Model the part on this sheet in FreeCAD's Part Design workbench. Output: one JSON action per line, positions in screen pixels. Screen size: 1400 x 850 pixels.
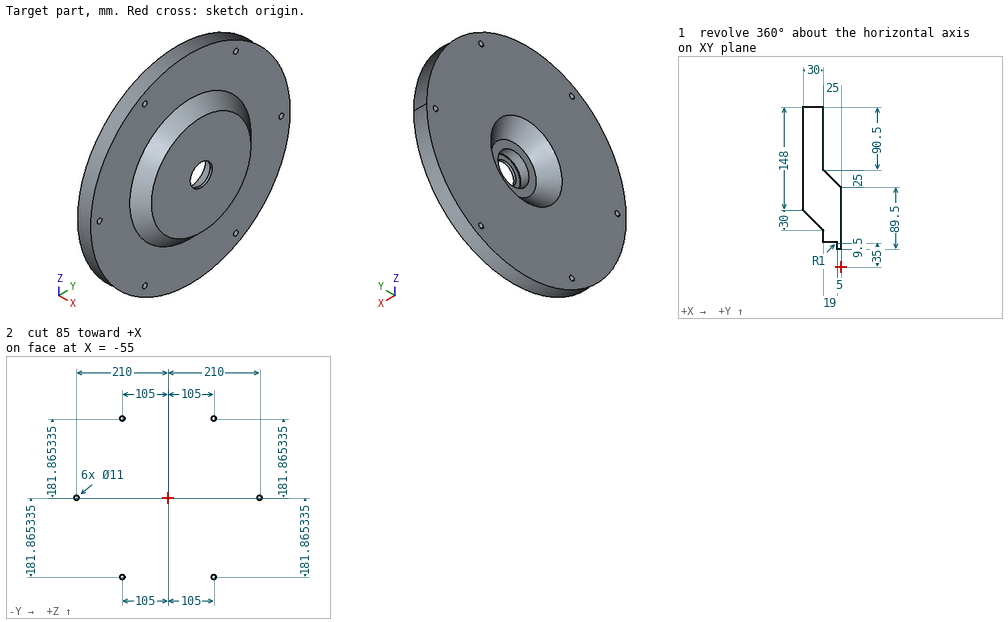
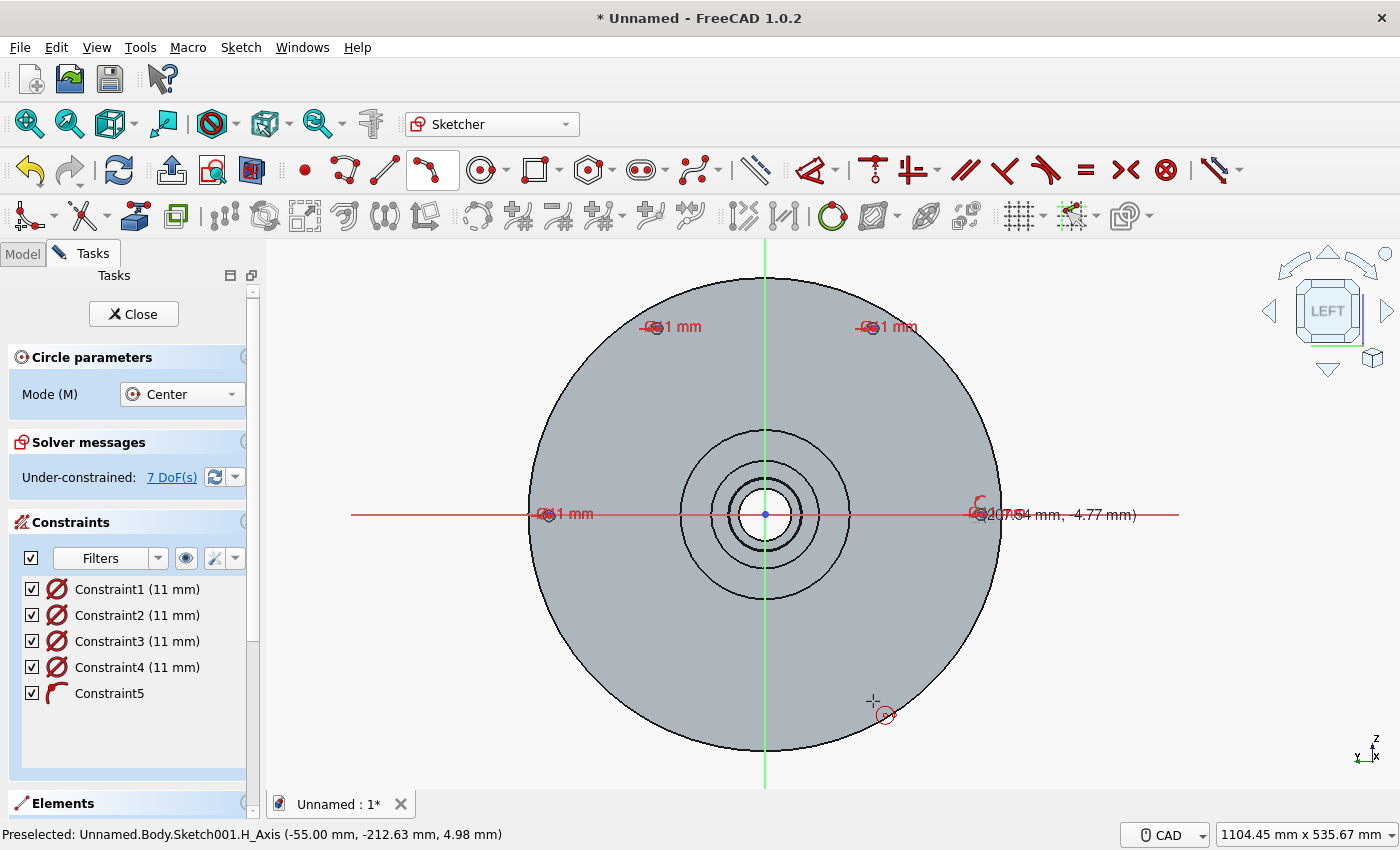
{"action": "left_click", "coordinate": [873, 701]}
{"action": "mouse_move", "coordinate": [877, 697]}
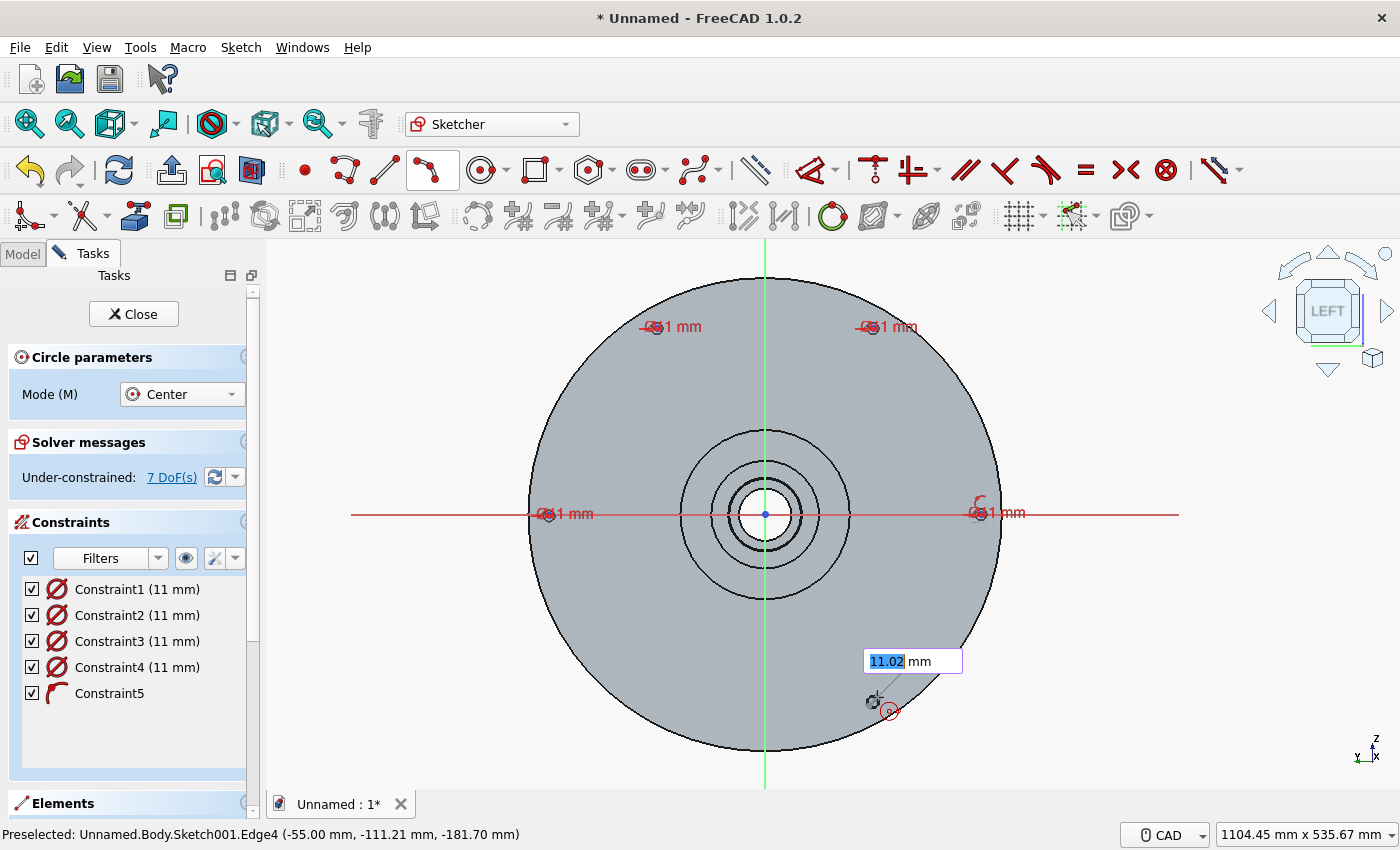
{"action": "type", "text": "11"}
{"action": "key", "text": "Return"}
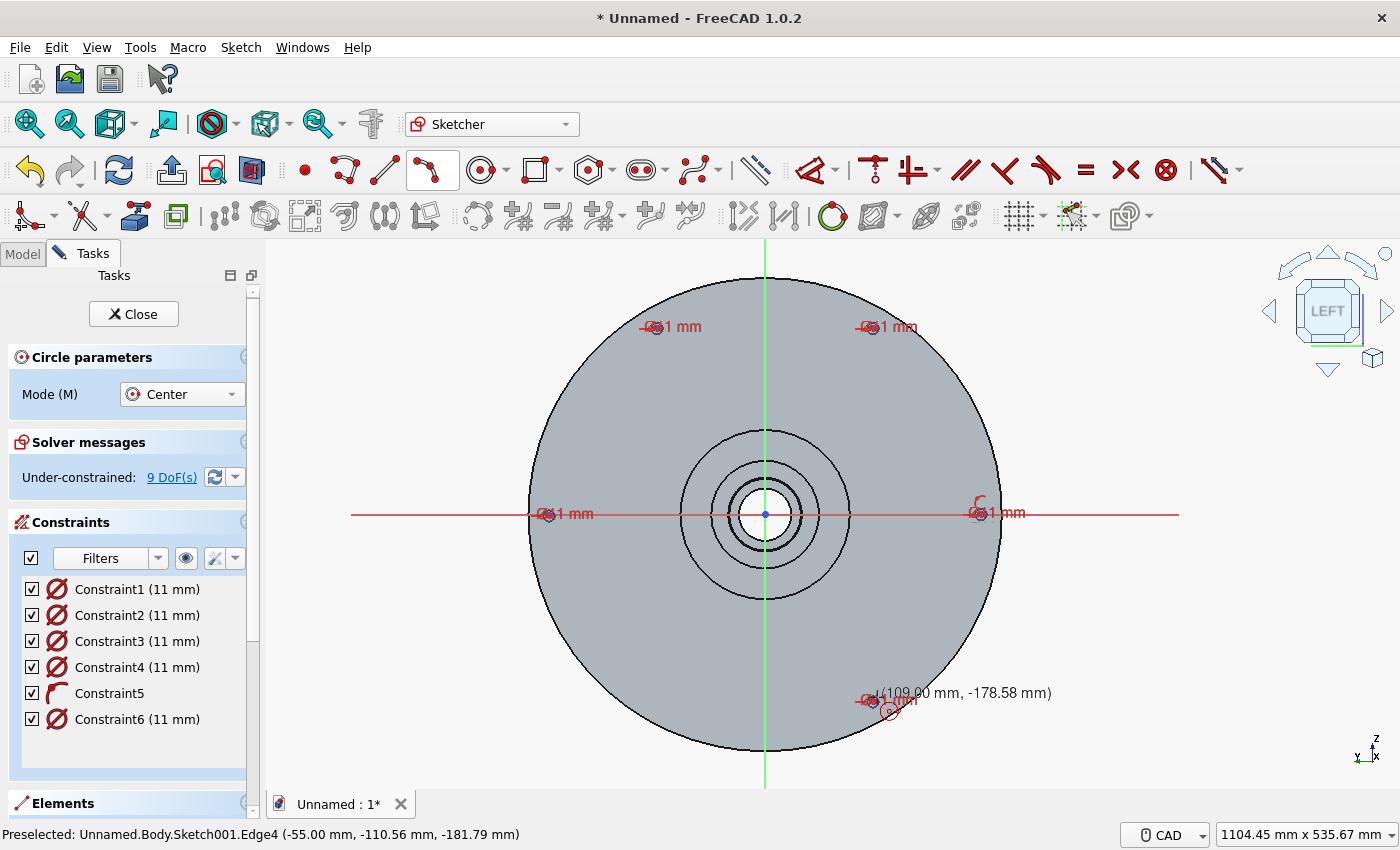
{"action": "scroll", "coordinate": [657, 701], "scroll_direction": "up", "scroll_amount": 7}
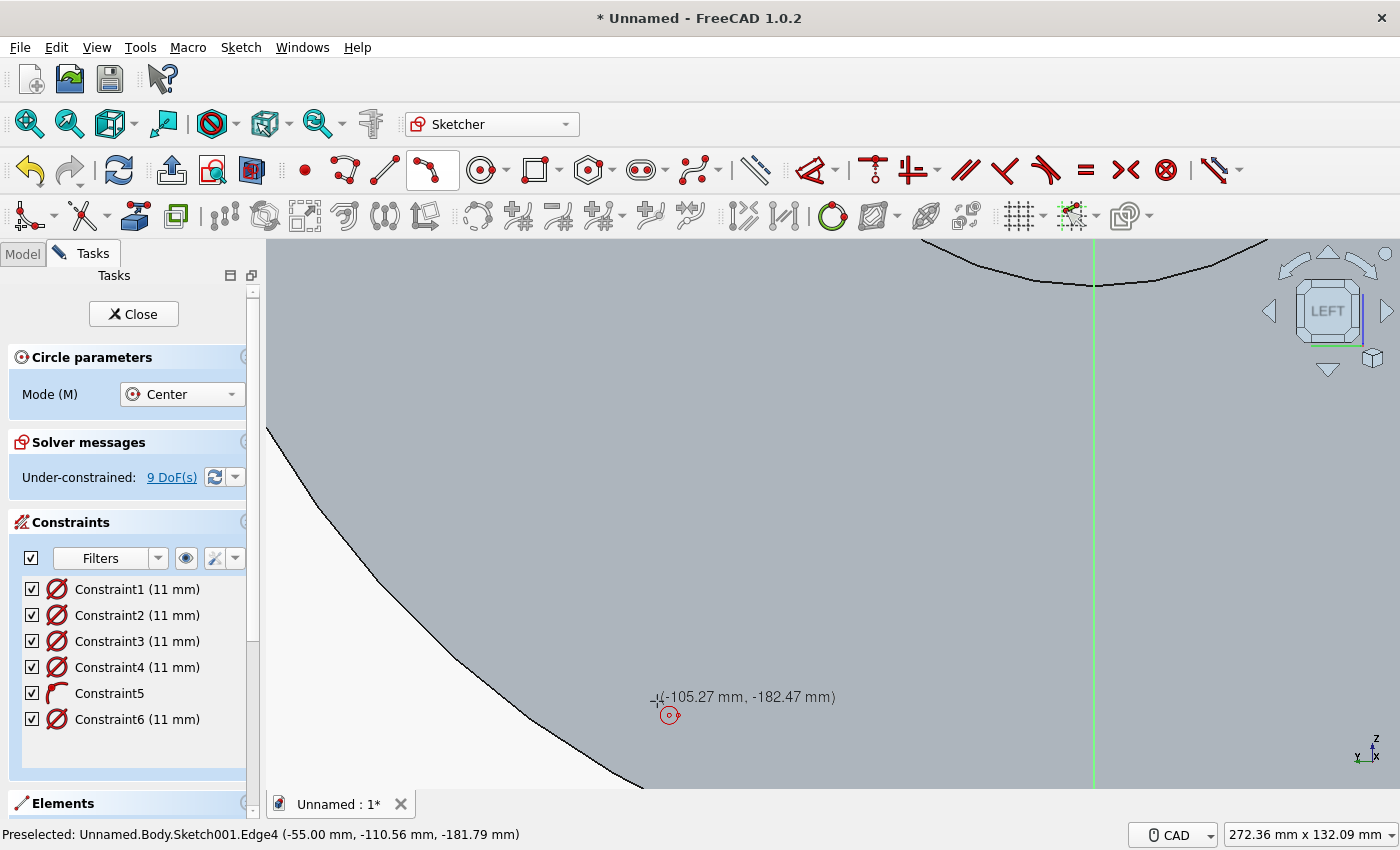
{"action": "scroll", "coordinate": [657, 701], "scroll_direction": "down", "scroll_amount": 7}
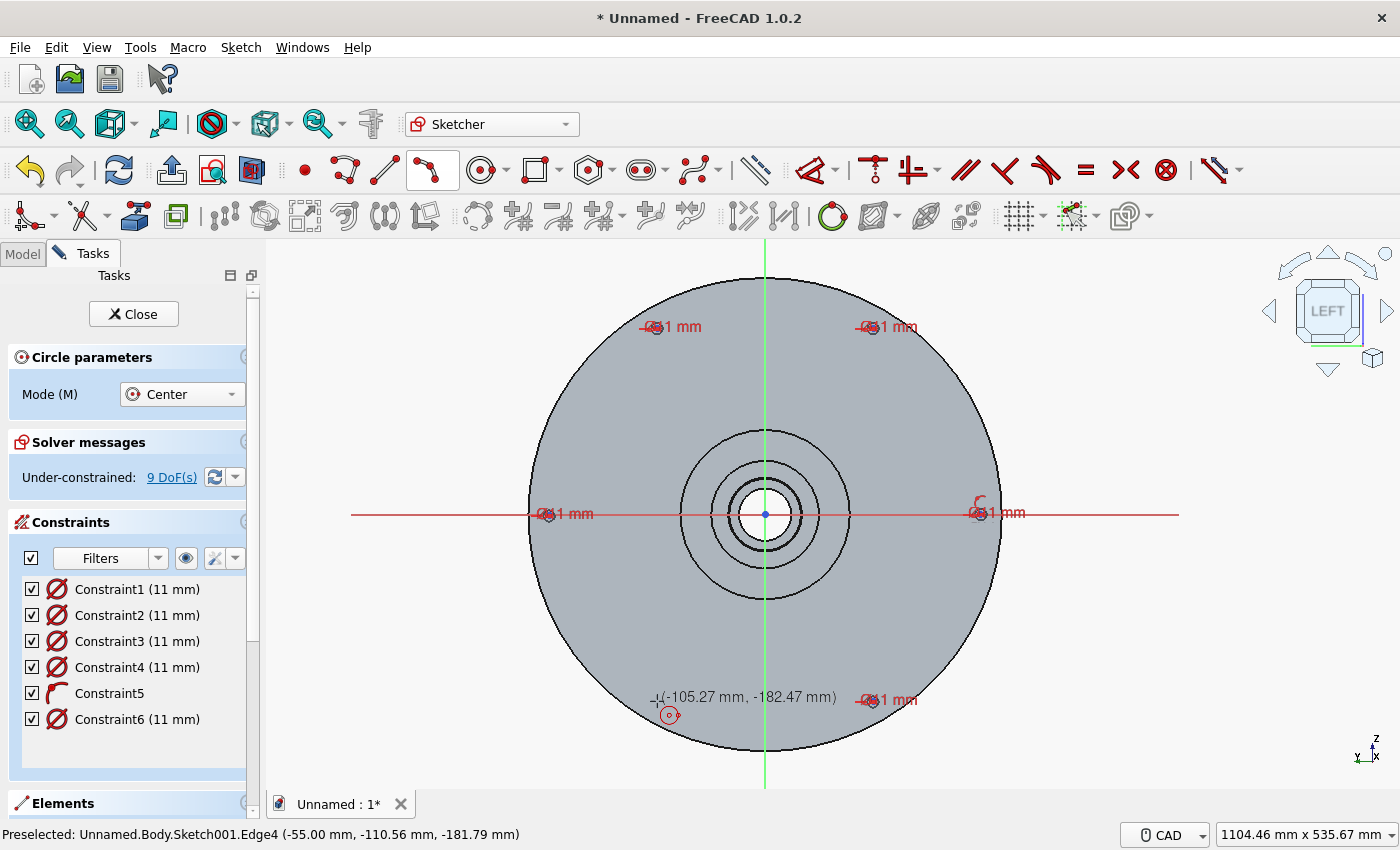
{"action": "left_click", "coordinate": [657, 701]}
{"action": "mouse_move", "coordinate": [661, 697]}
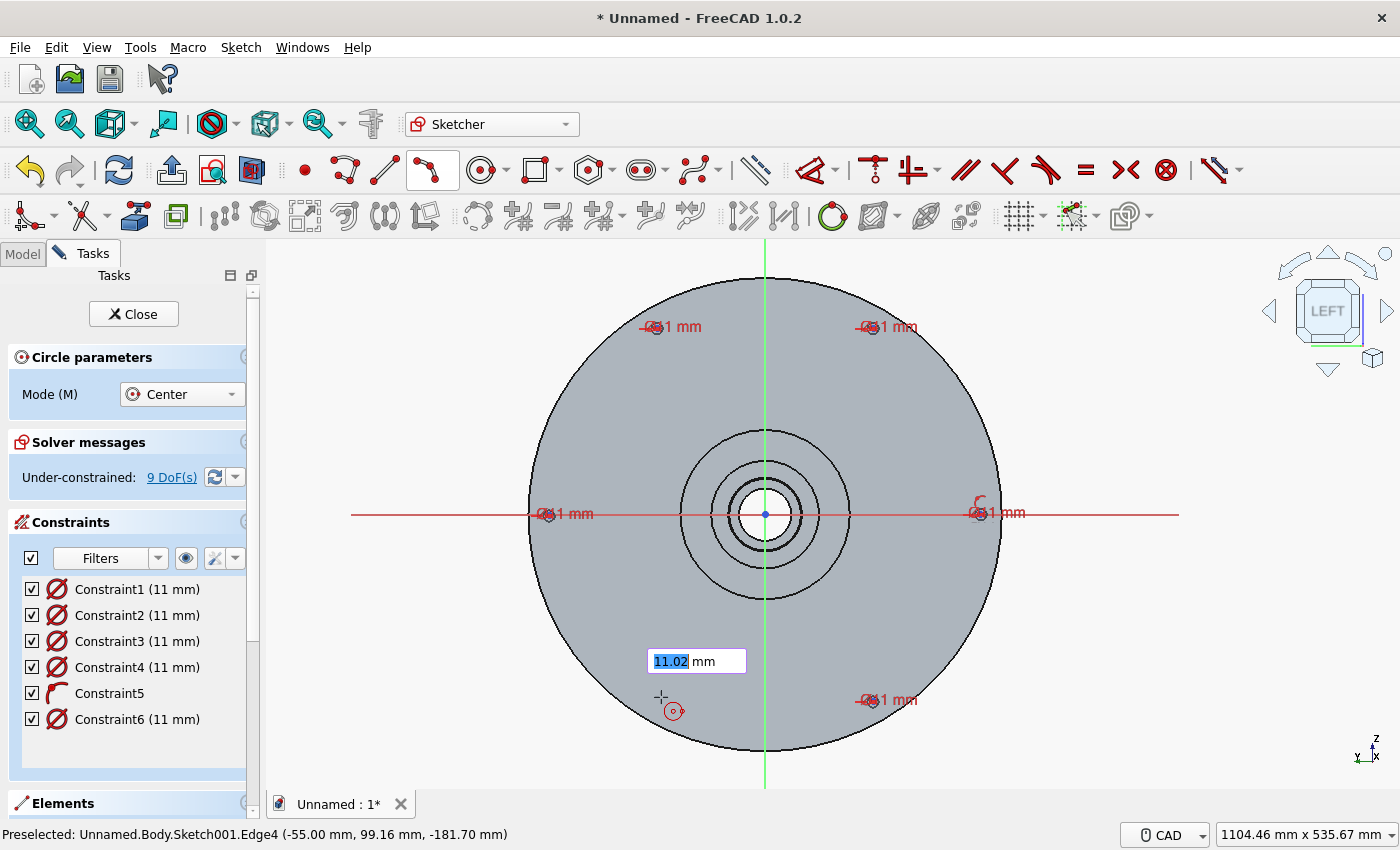
{"action": "type", "text": "11"}
{"action": "key", "text": "Return"}
{"action": "key", "text": "Escape"}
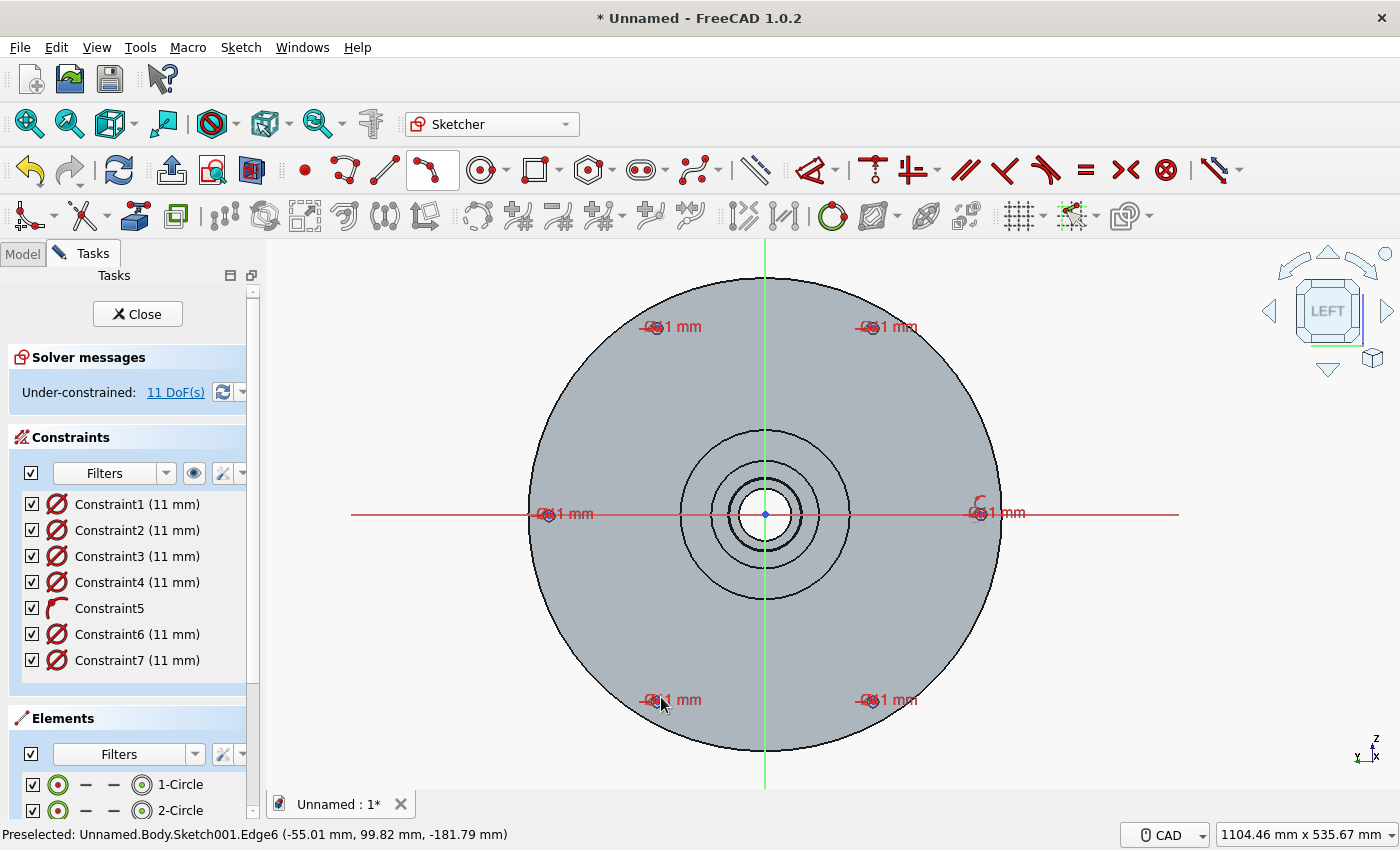
{"action": "left_click", "coordinate": [549, 516]}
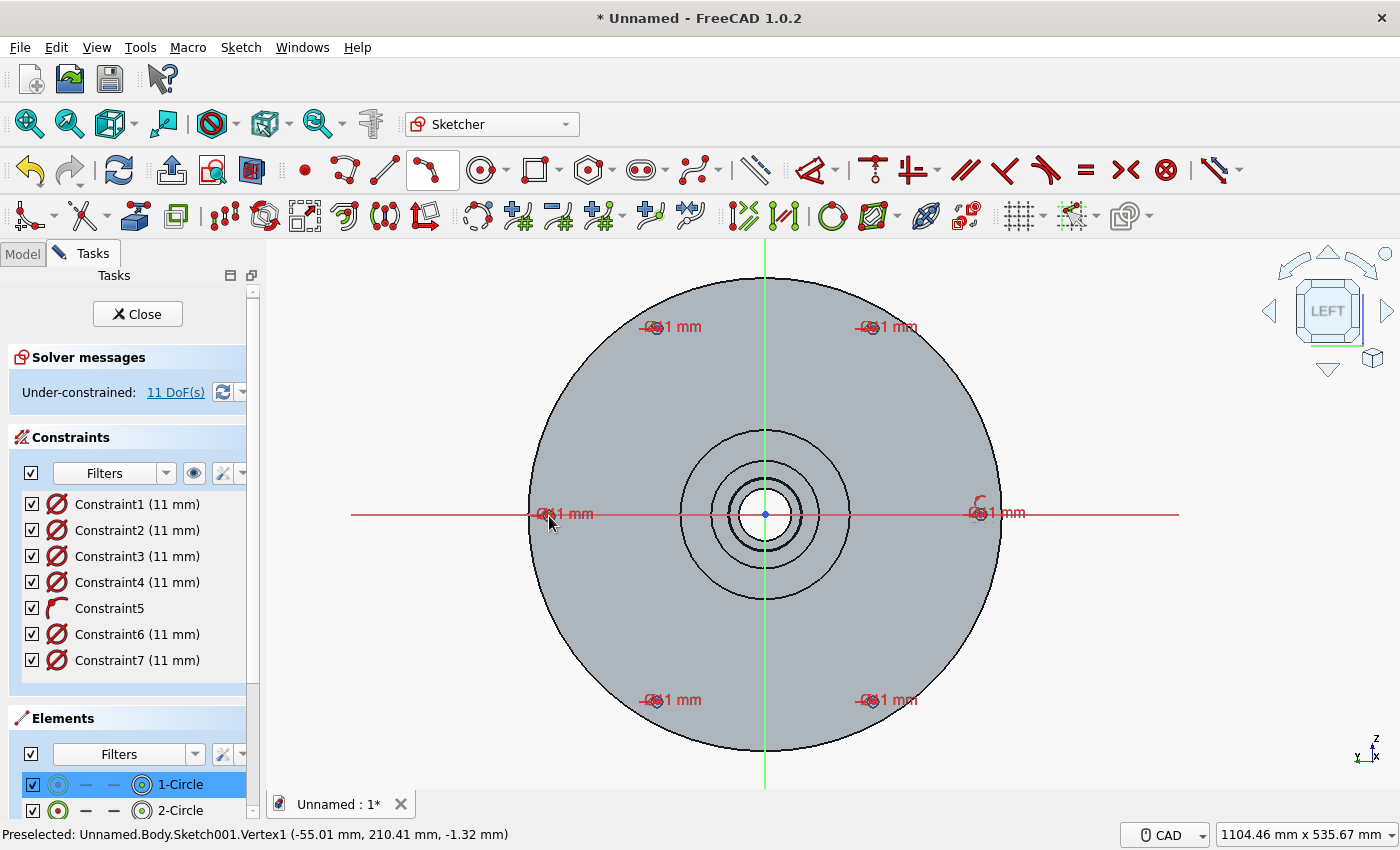
{"action": "left_click", "coordinate": [361, 515]}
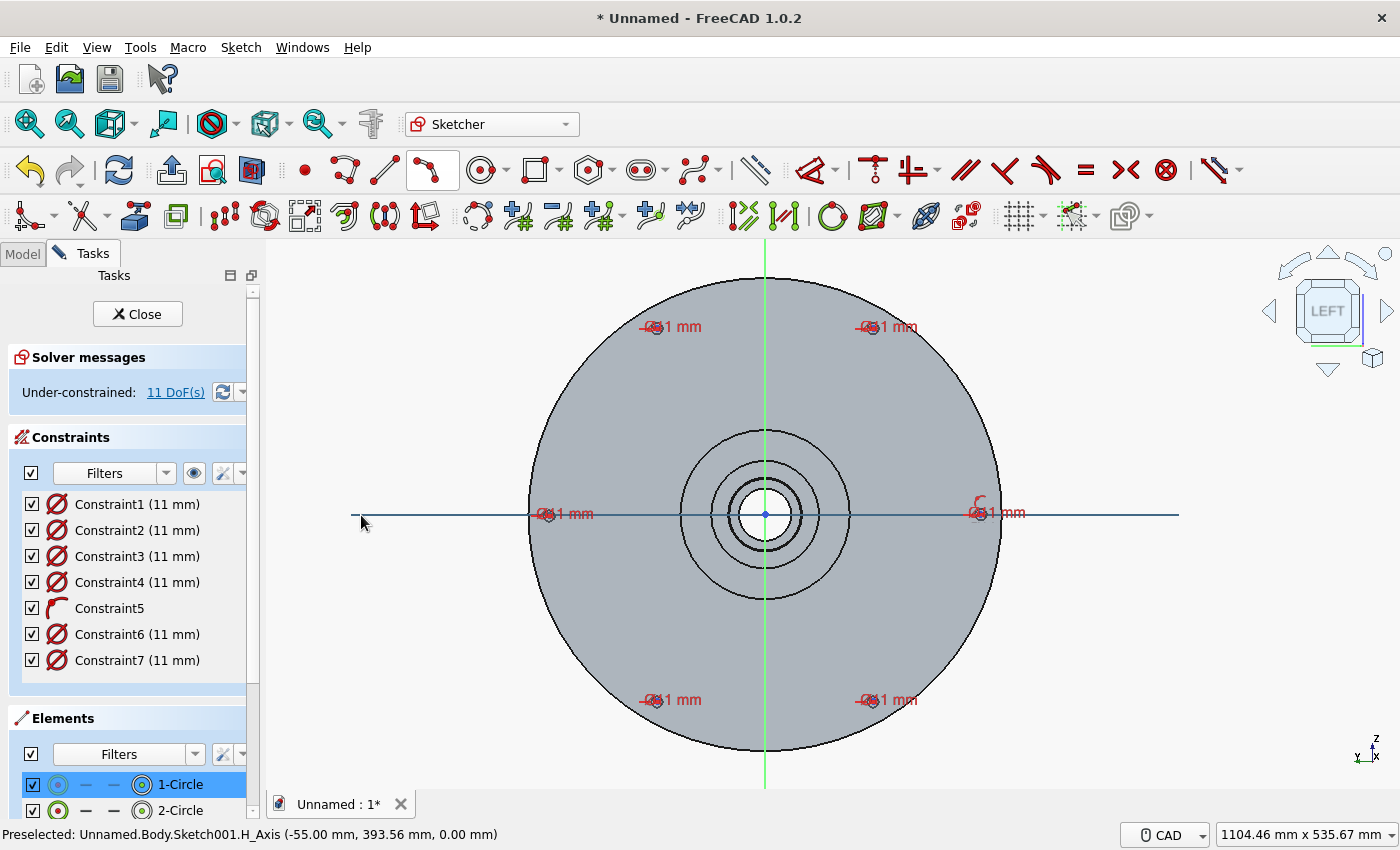
{"action": "left_click", "coordinate": [874, 170]}